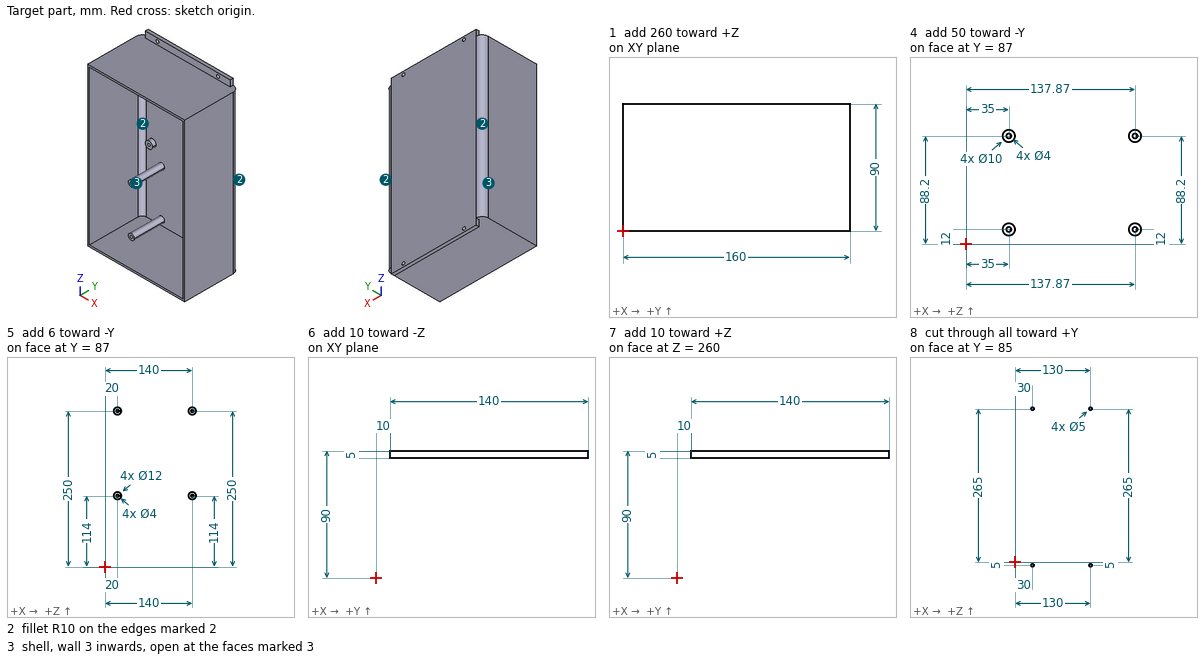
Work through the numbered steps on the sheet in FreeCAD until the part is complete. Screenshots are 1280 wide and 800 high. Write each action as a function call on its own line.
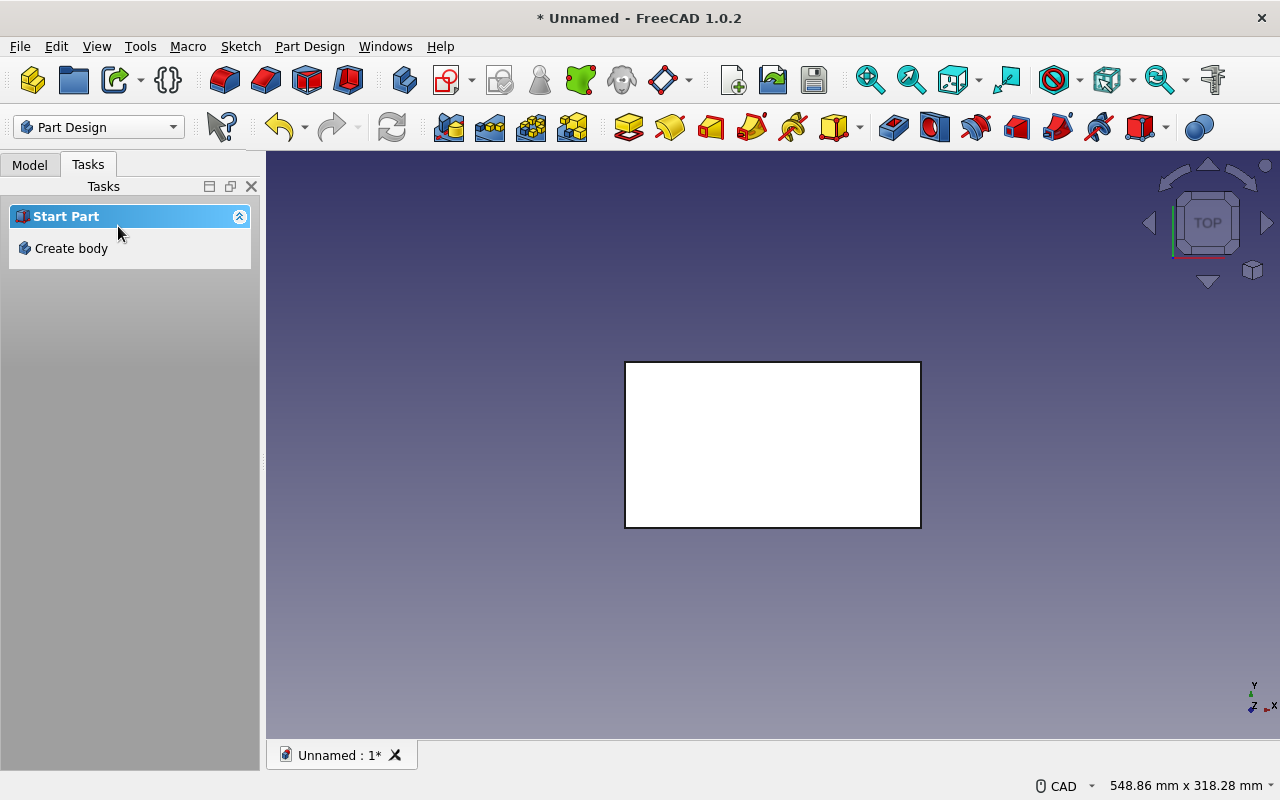
key(1)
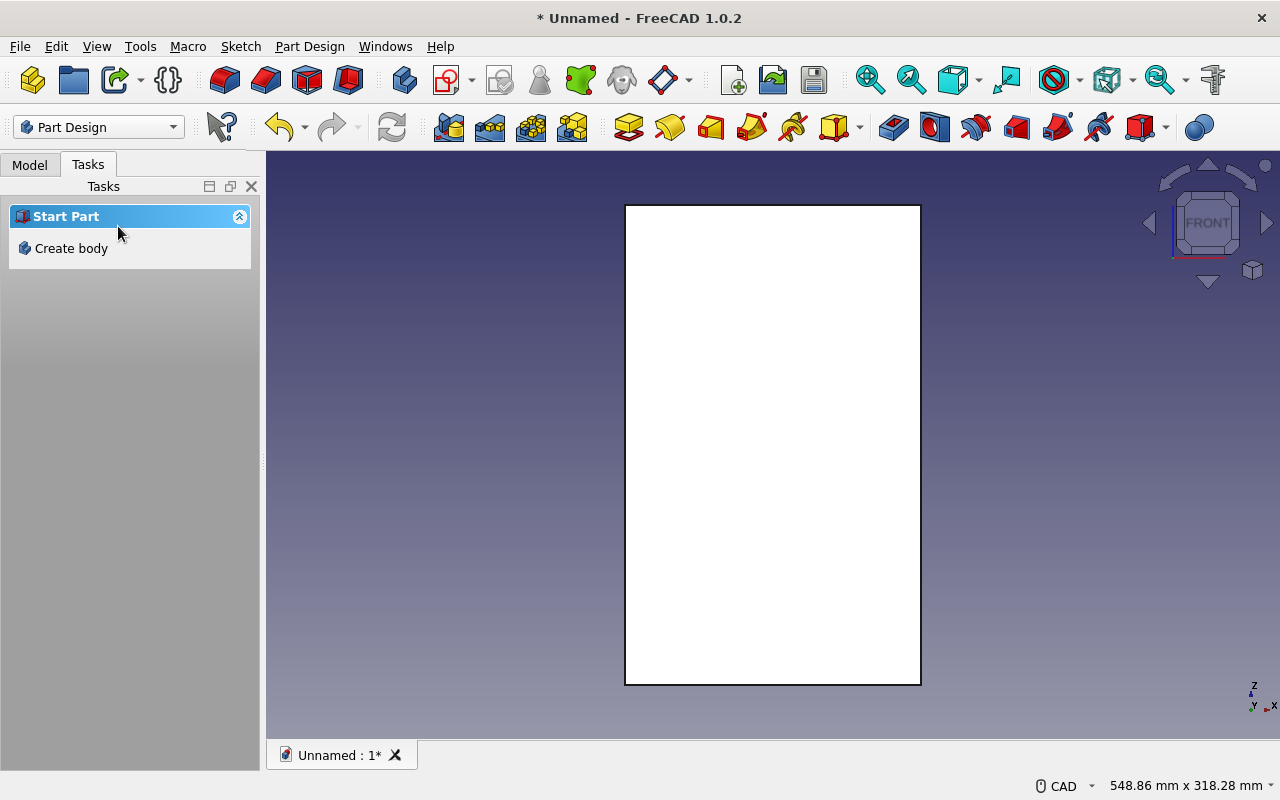
key(3)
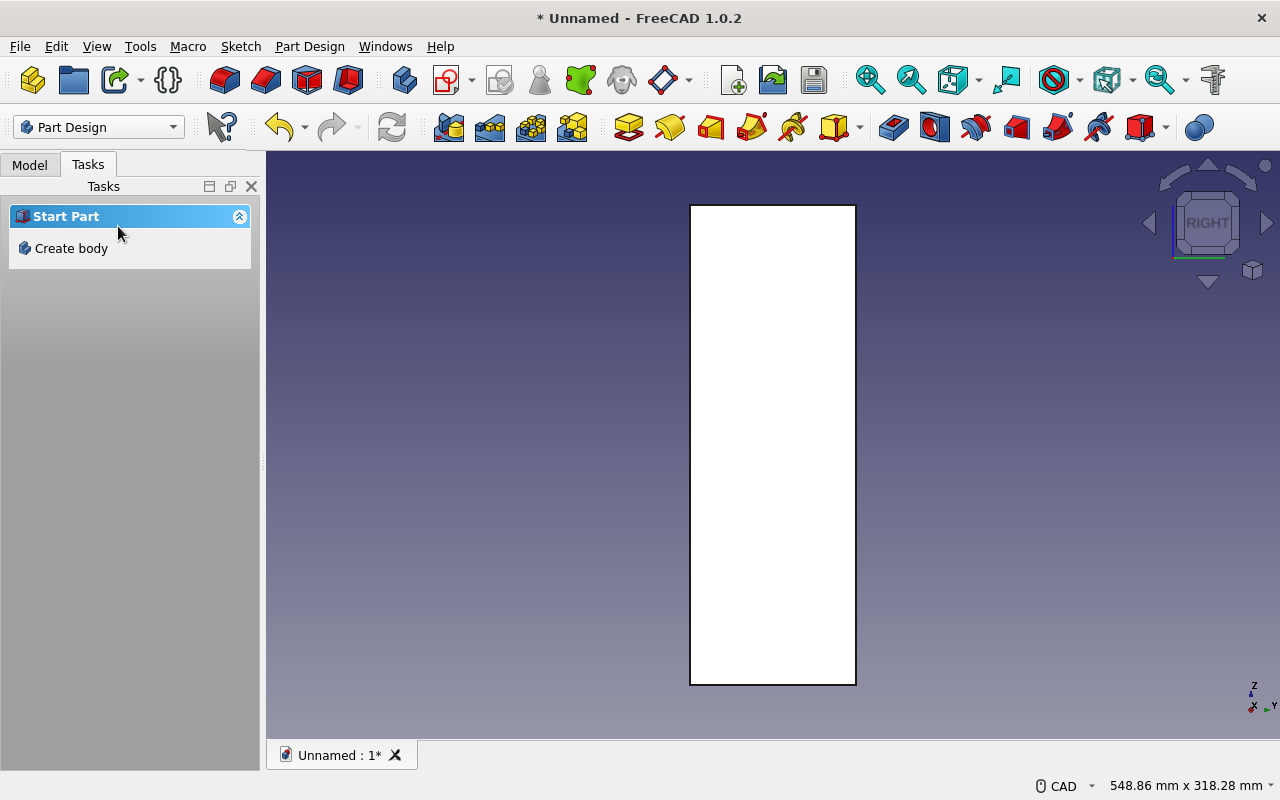
click(856, 444)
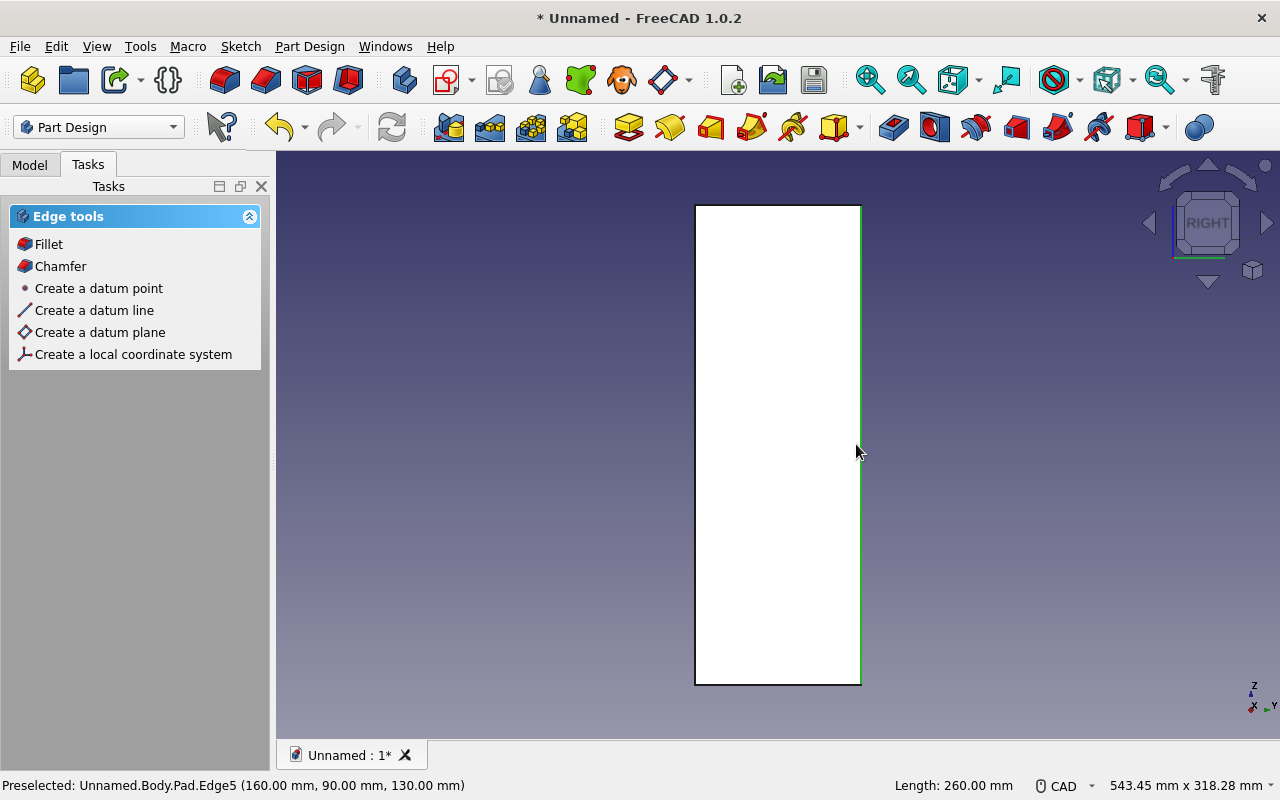
key(5)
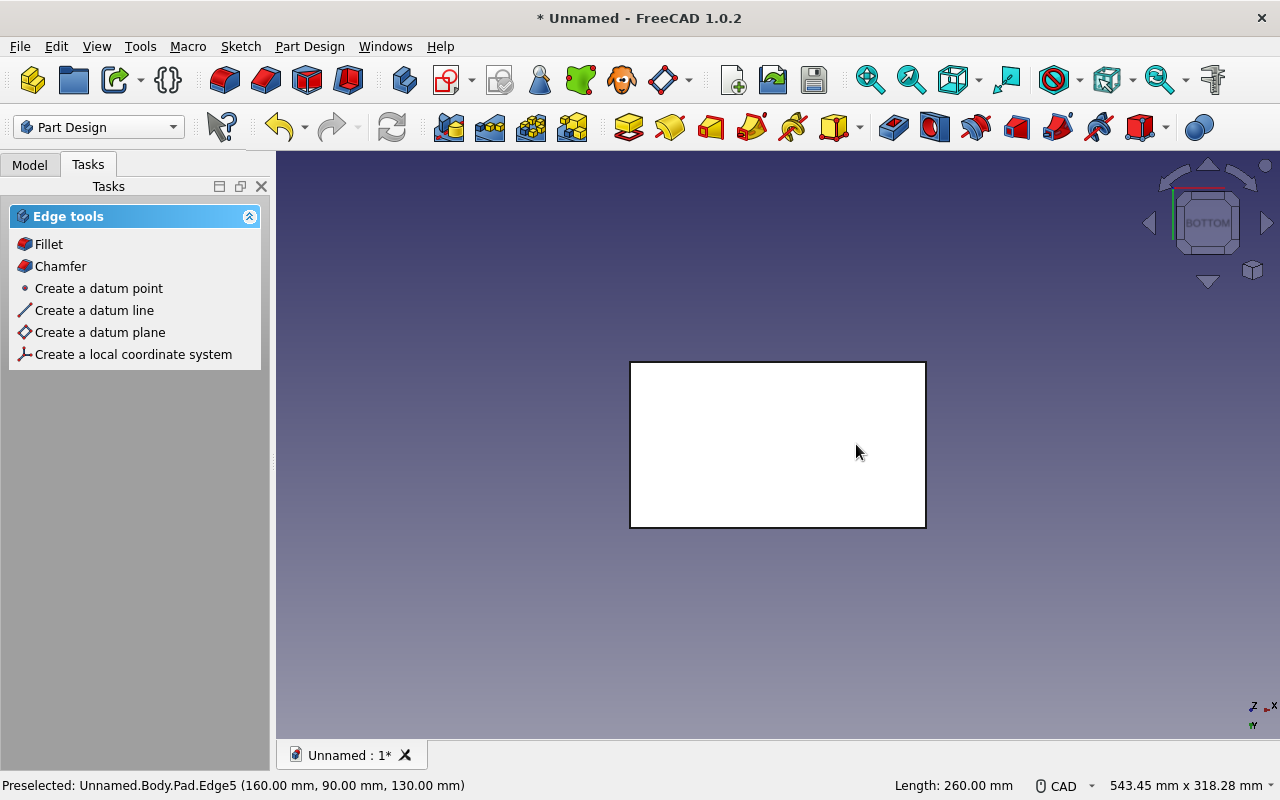
click(871, 80)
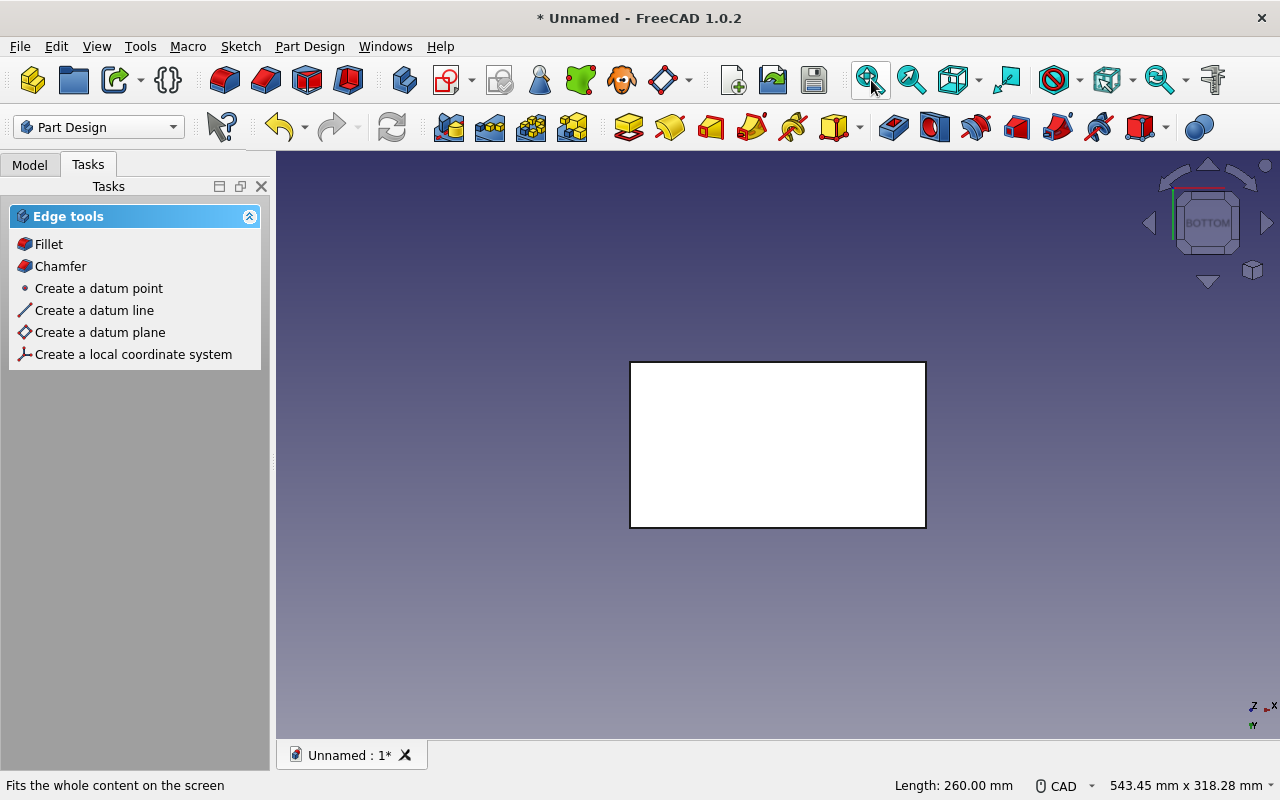
key(4)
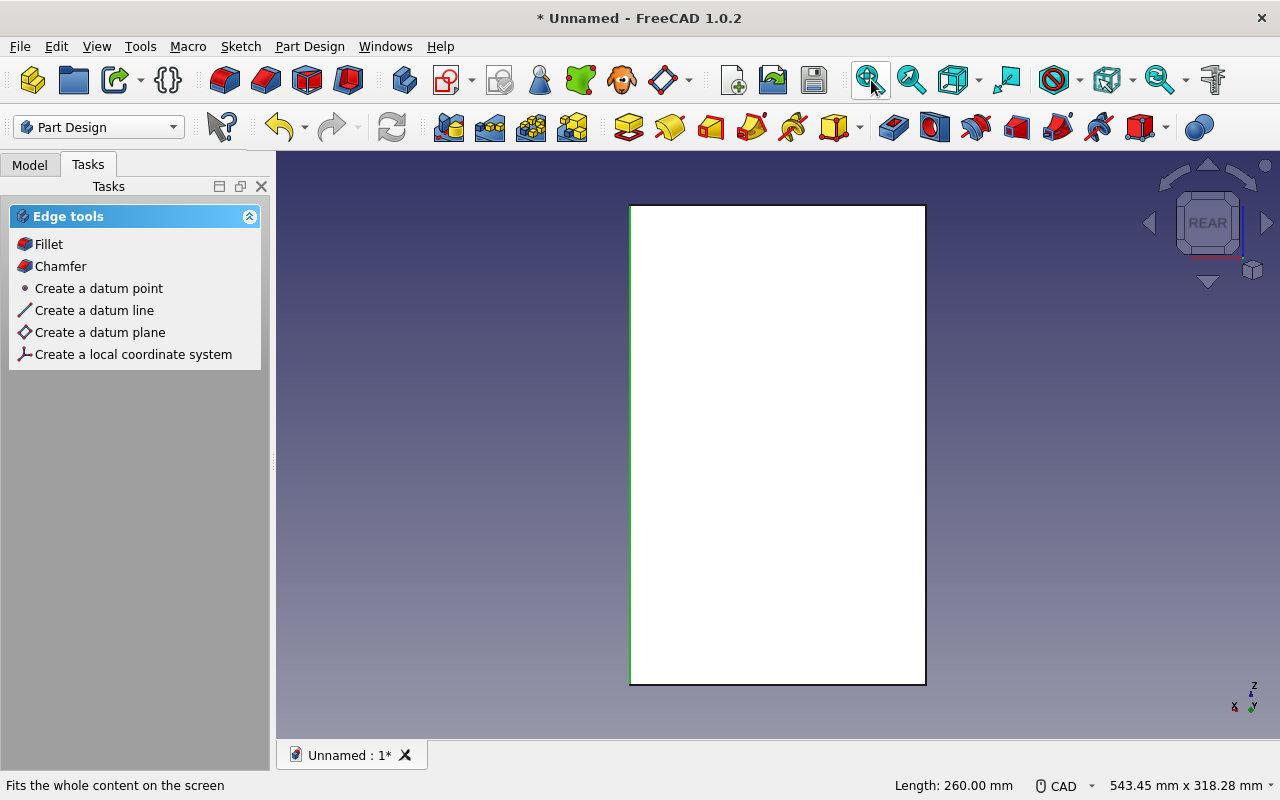
click(926, 444, ctrl)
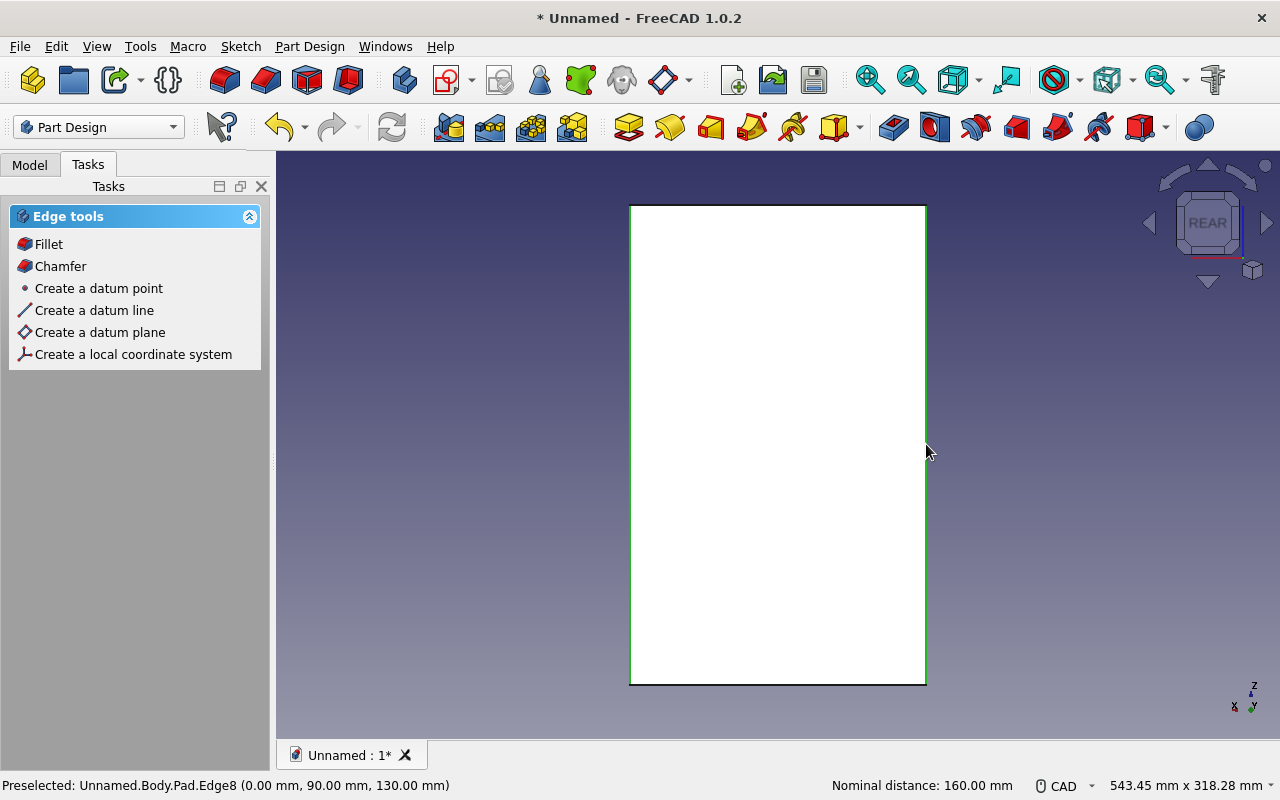
click(225, 80)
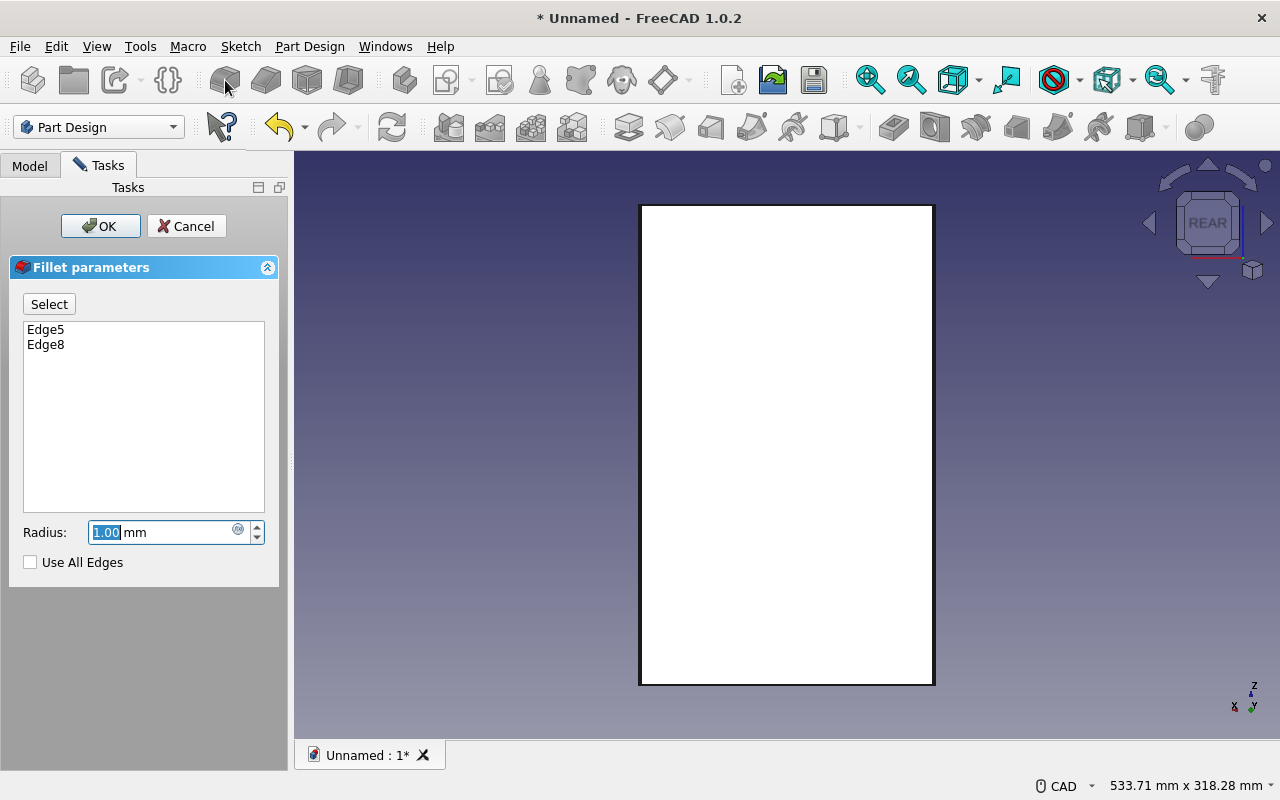
text(10)
key(Tab)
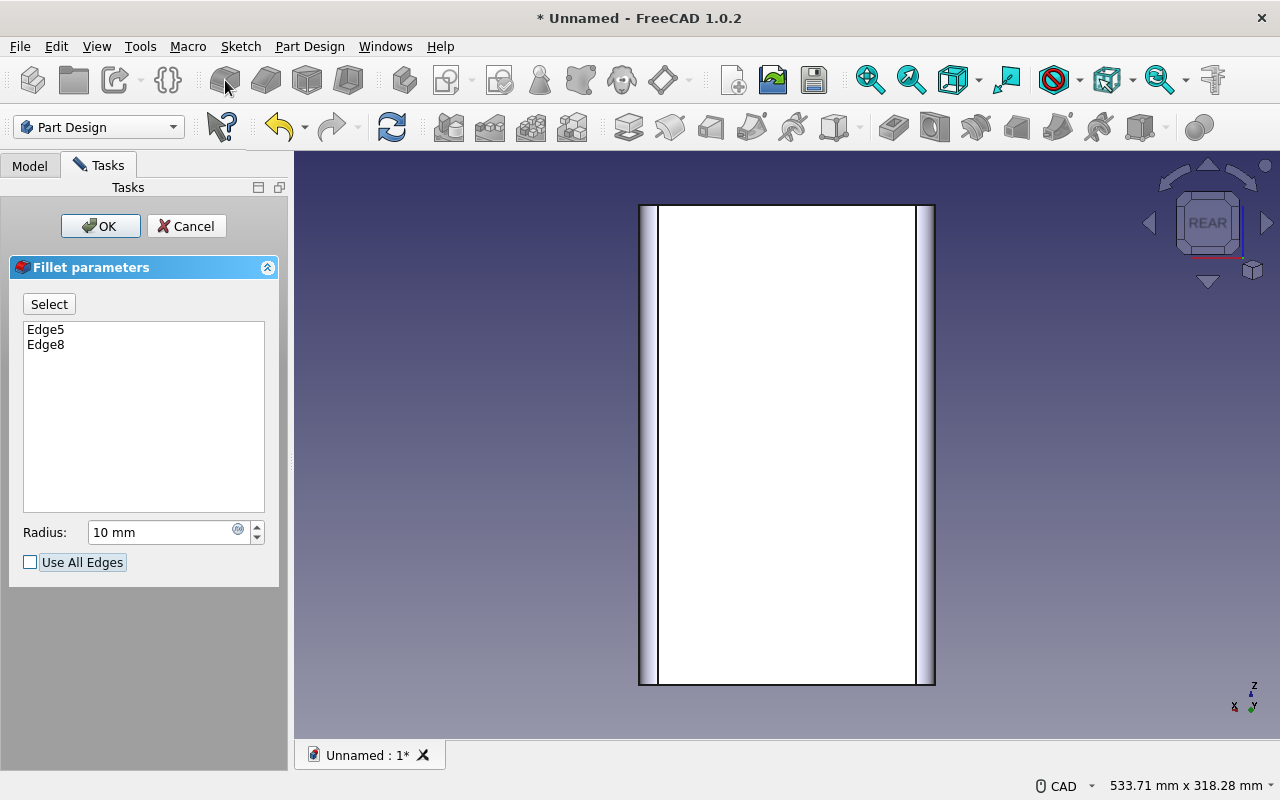
click(101, 226)